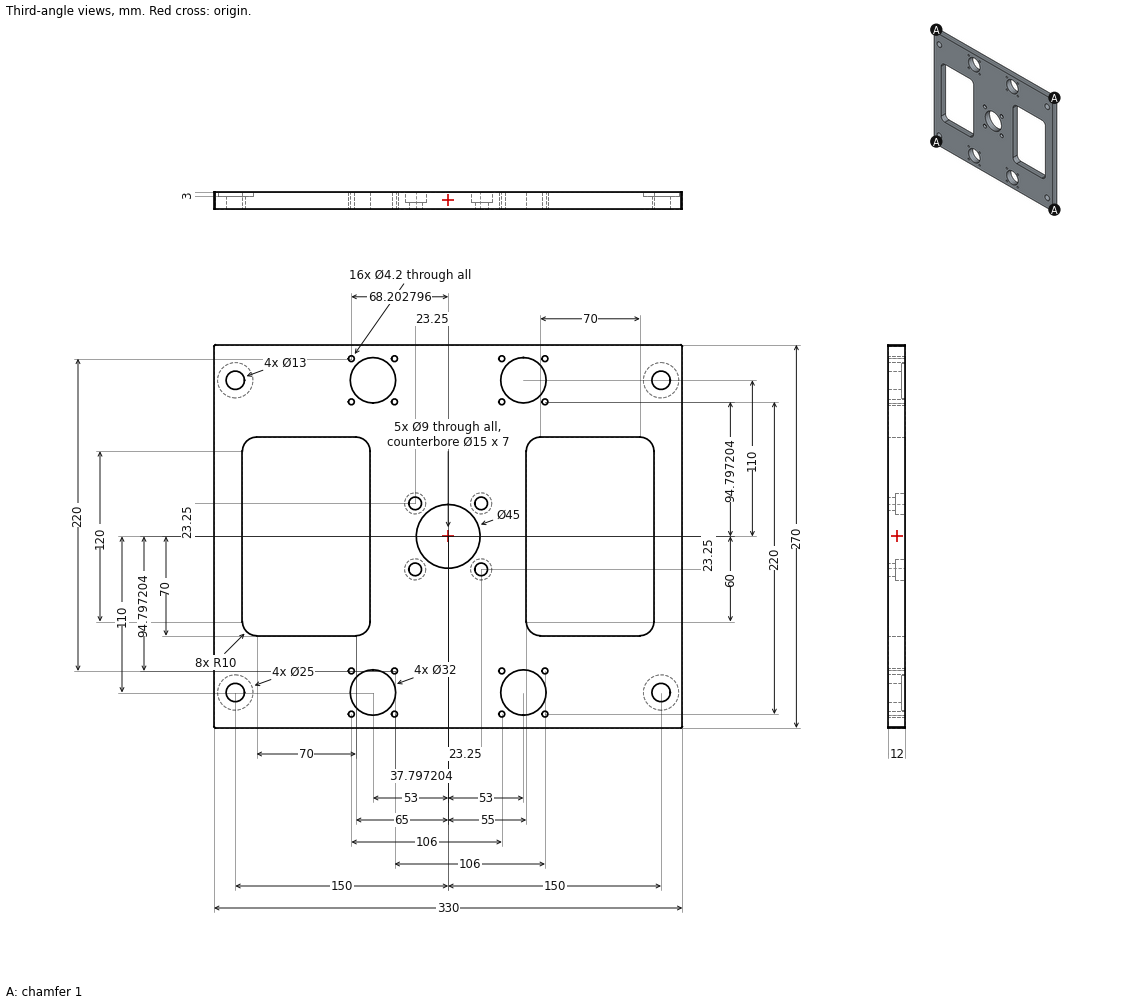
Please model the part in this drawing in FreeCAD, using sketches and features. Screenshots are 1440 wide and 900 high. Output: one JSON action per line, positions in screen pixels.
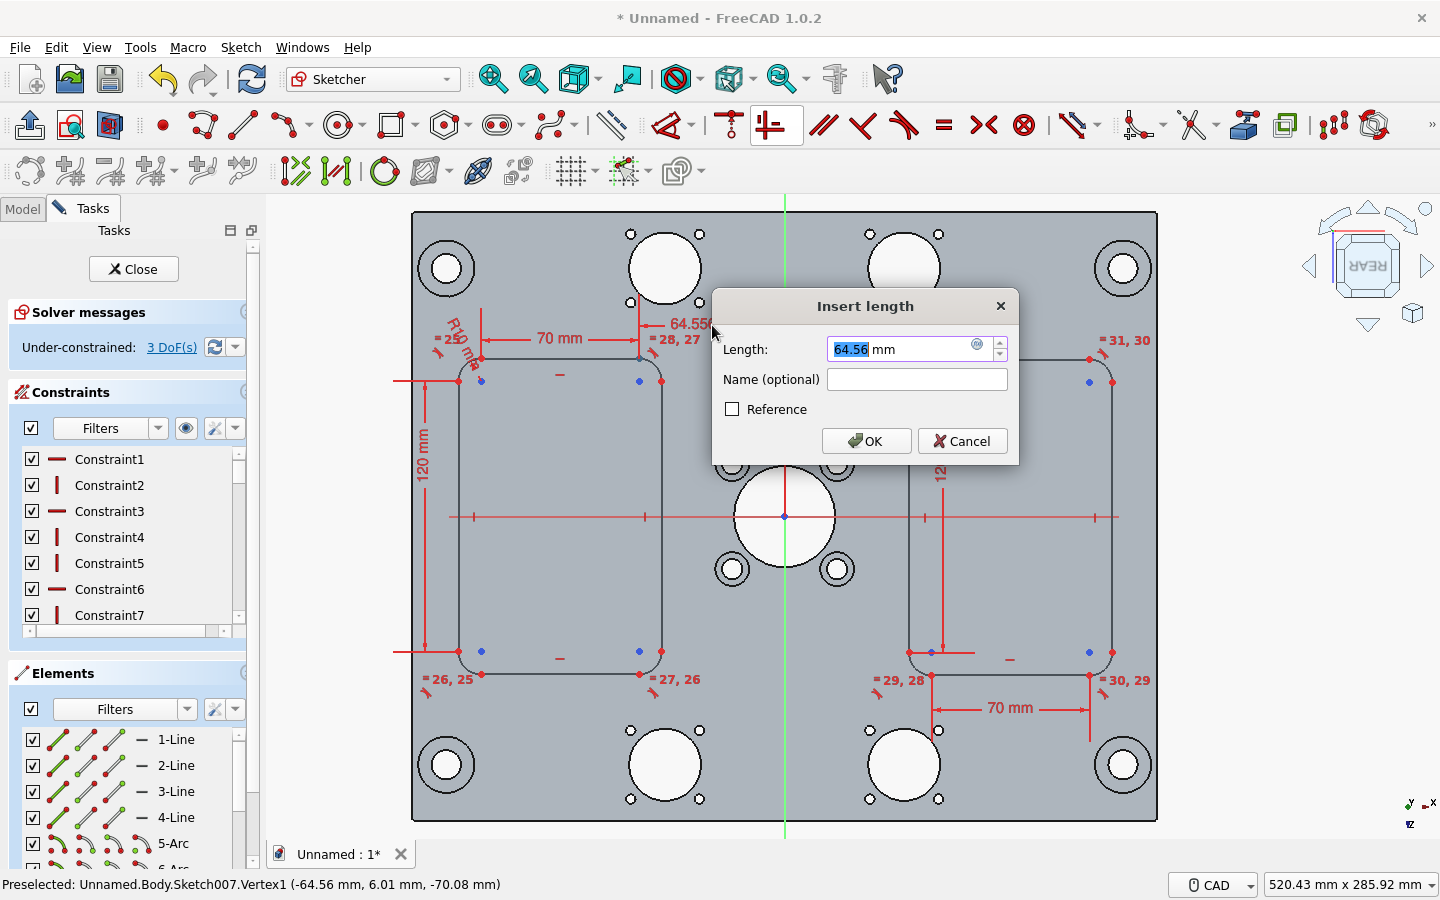
{"action": "type", "text": "65"}
{"action": "key", "text": "Return"}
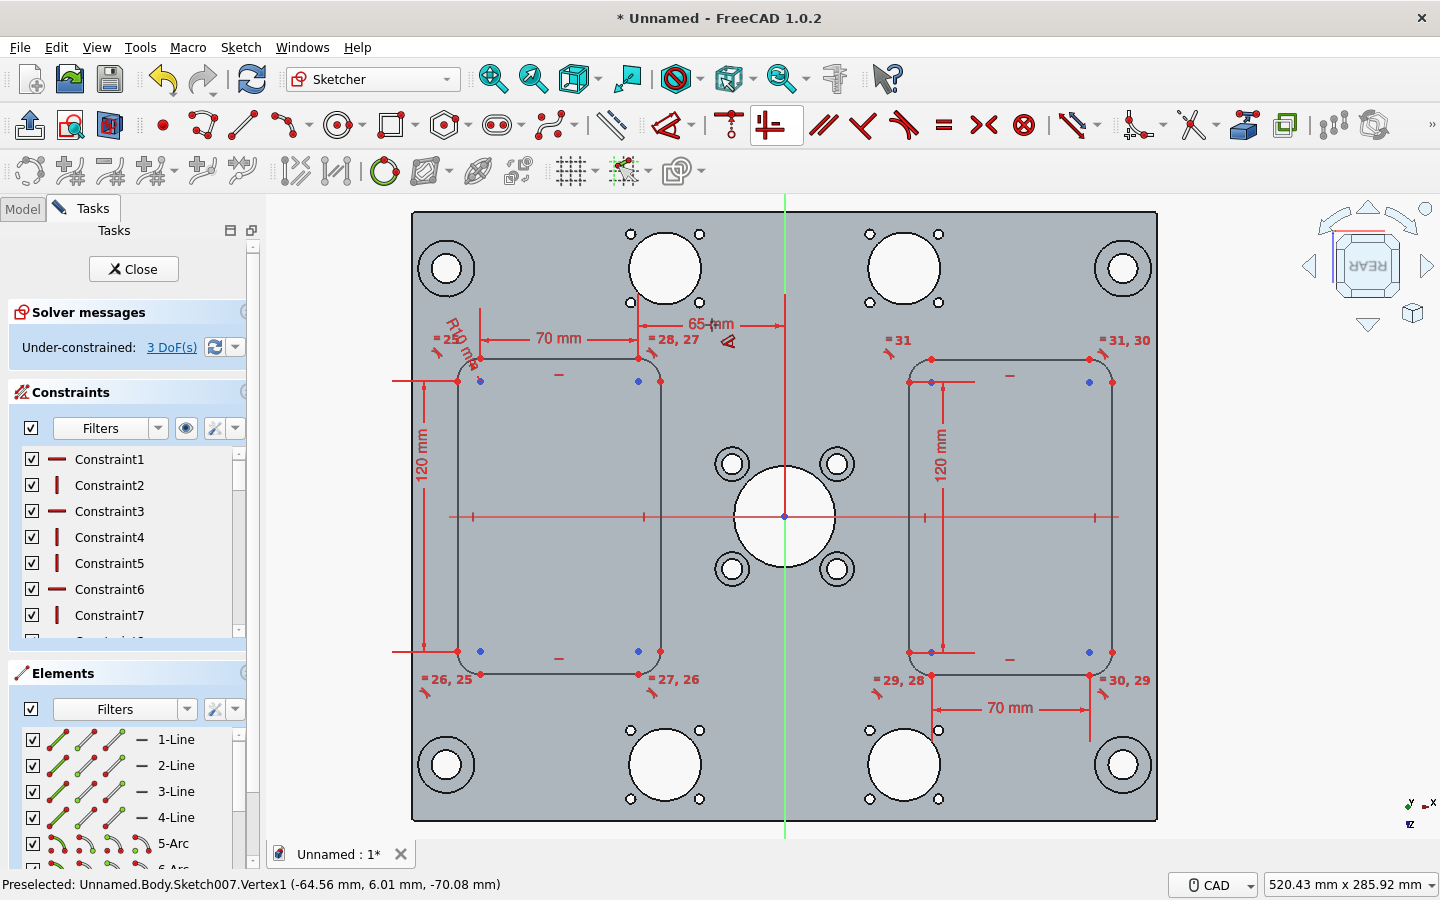
{"action": "left_click", "coordinate": [638, 359]}
{"action": "left_click", "coordinate": [604, 438]}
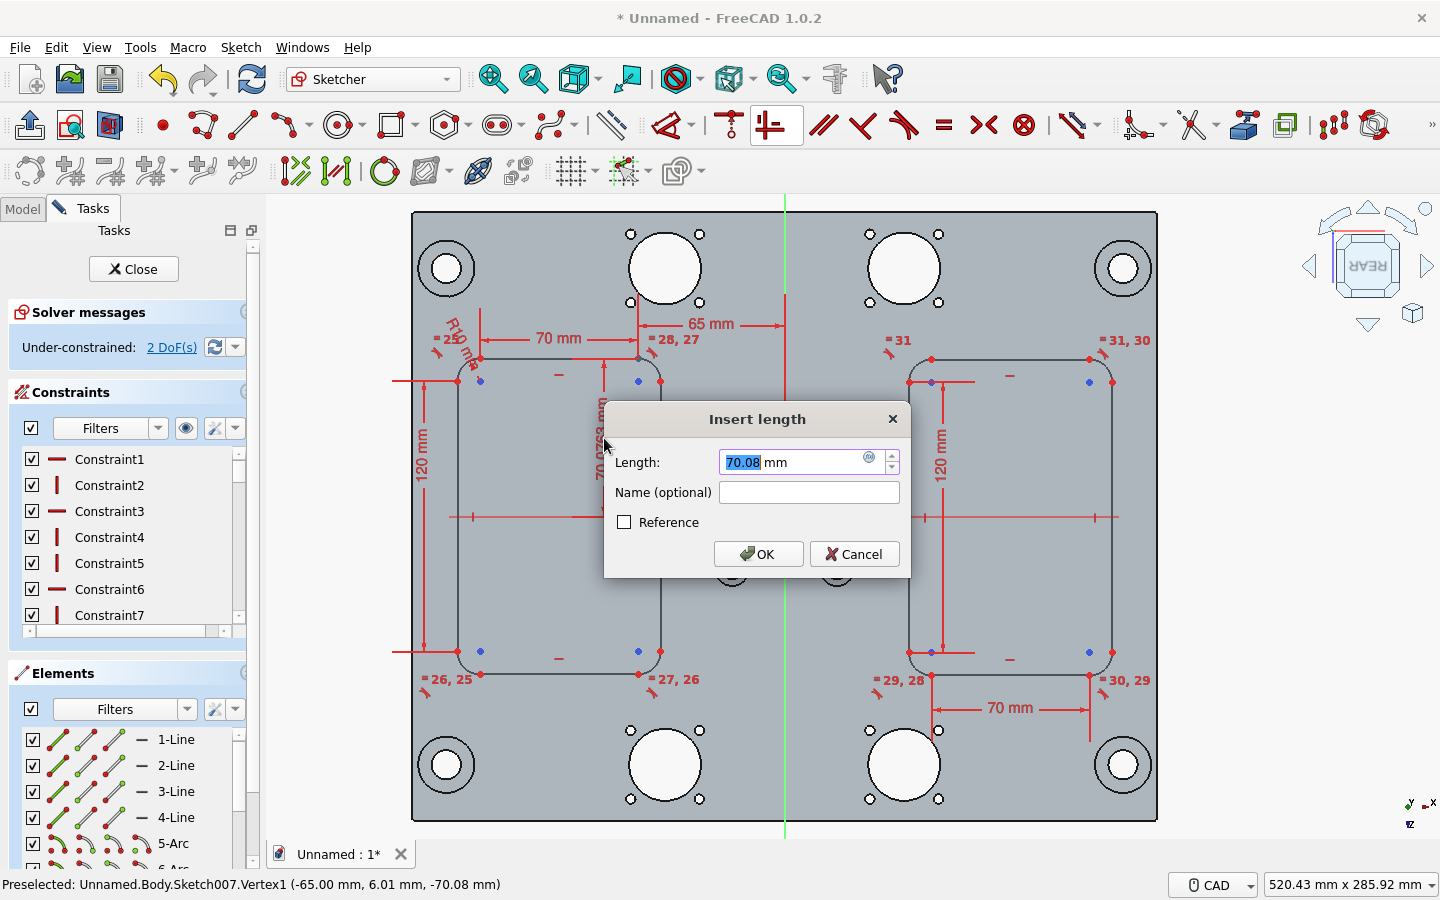
{"action": "type", "text": "70"}
{"action": "key", "text": "Return"}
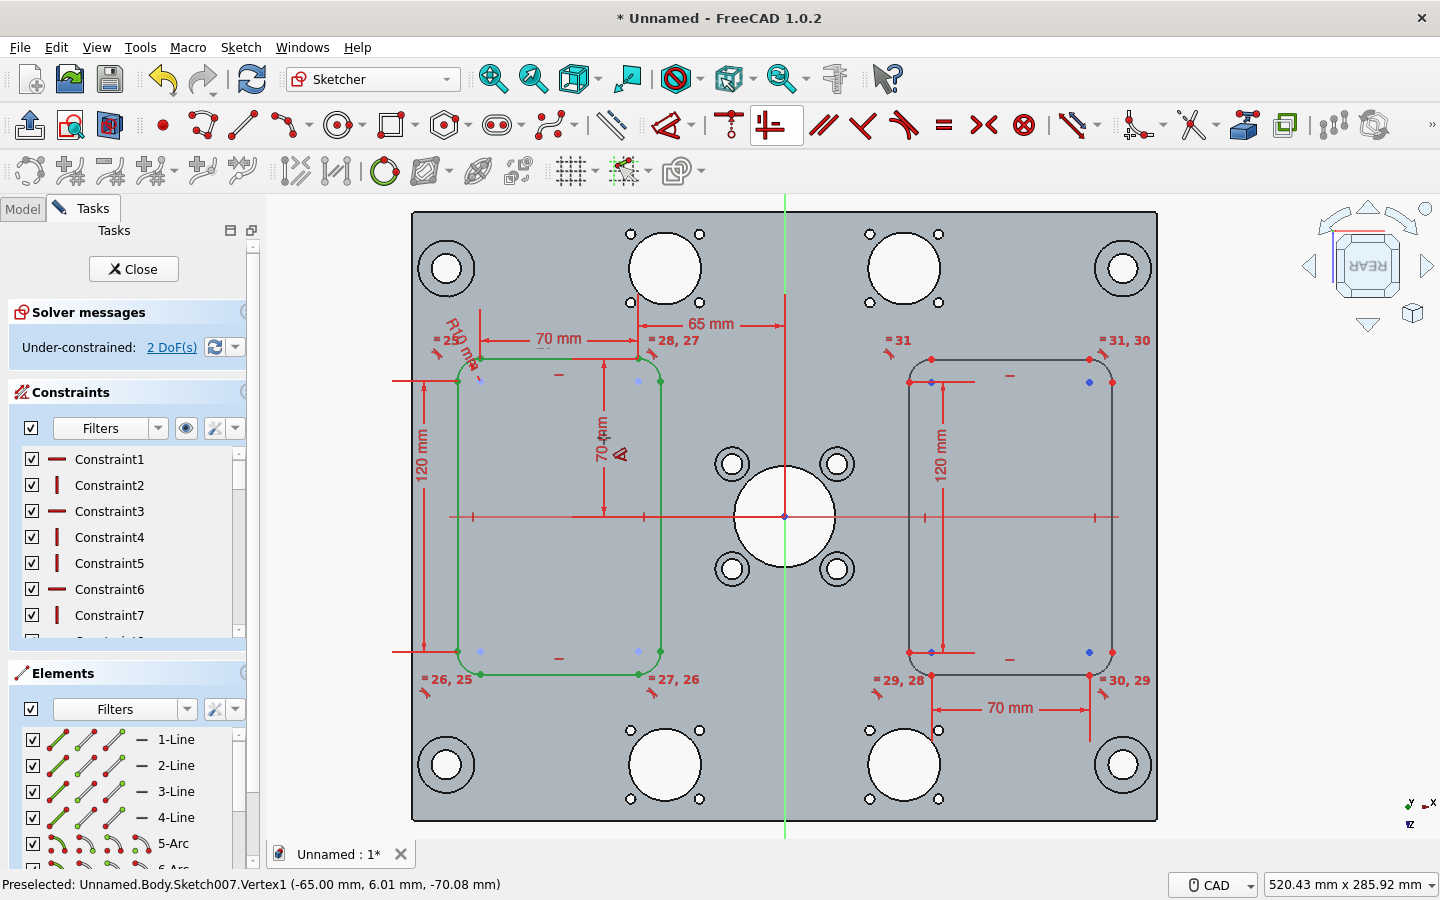
{"action": "left_click", "coordinate": [909, 382]}
{"action": "left_click", "coordinate": [847, 348]}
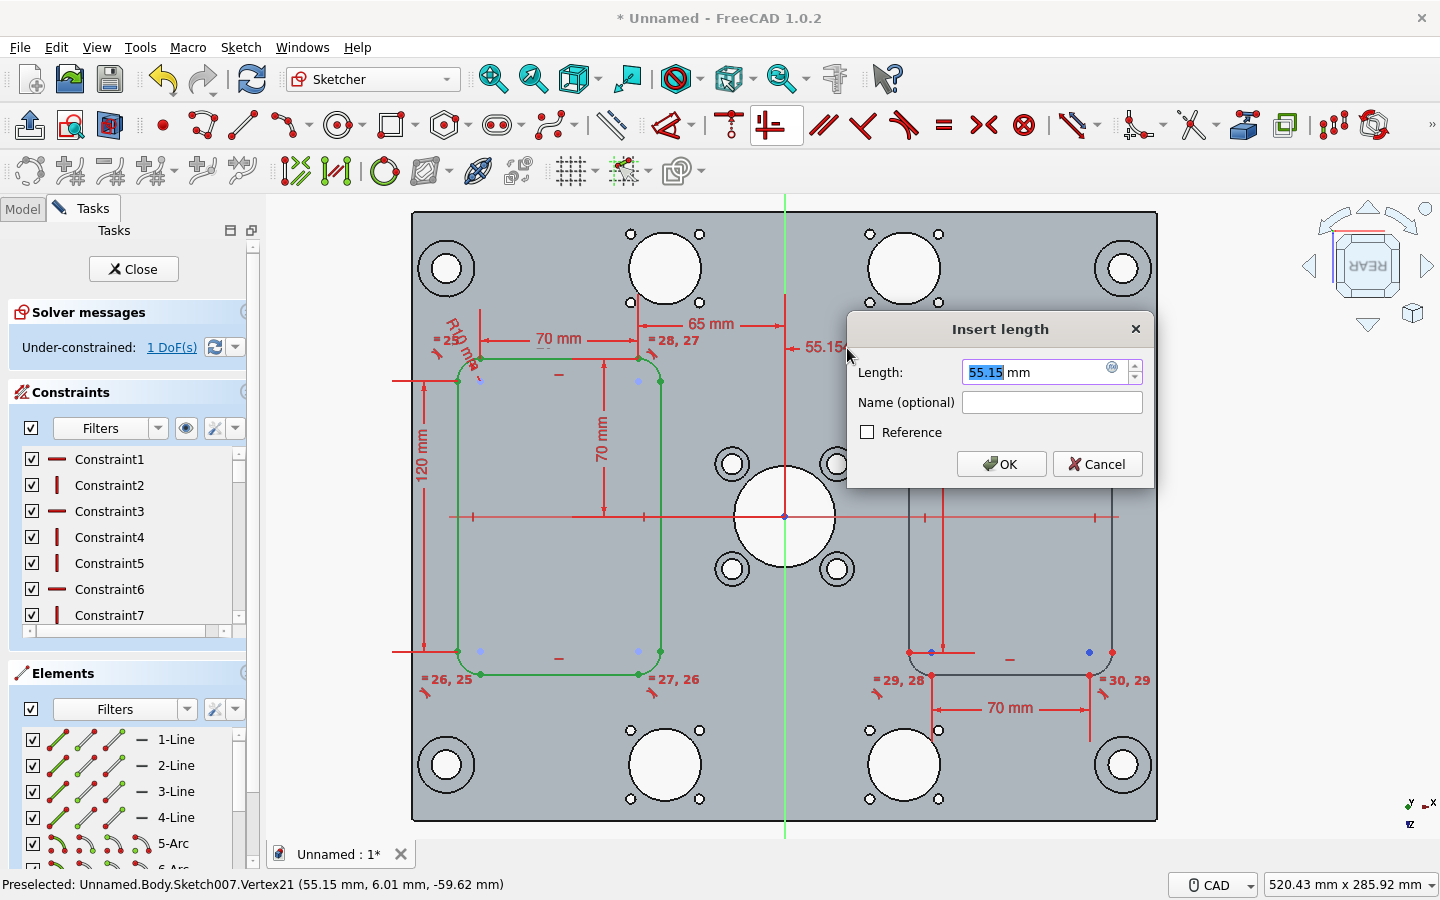
{"action": "type", "text": "55"}
{"action": "key", "text": "Return"}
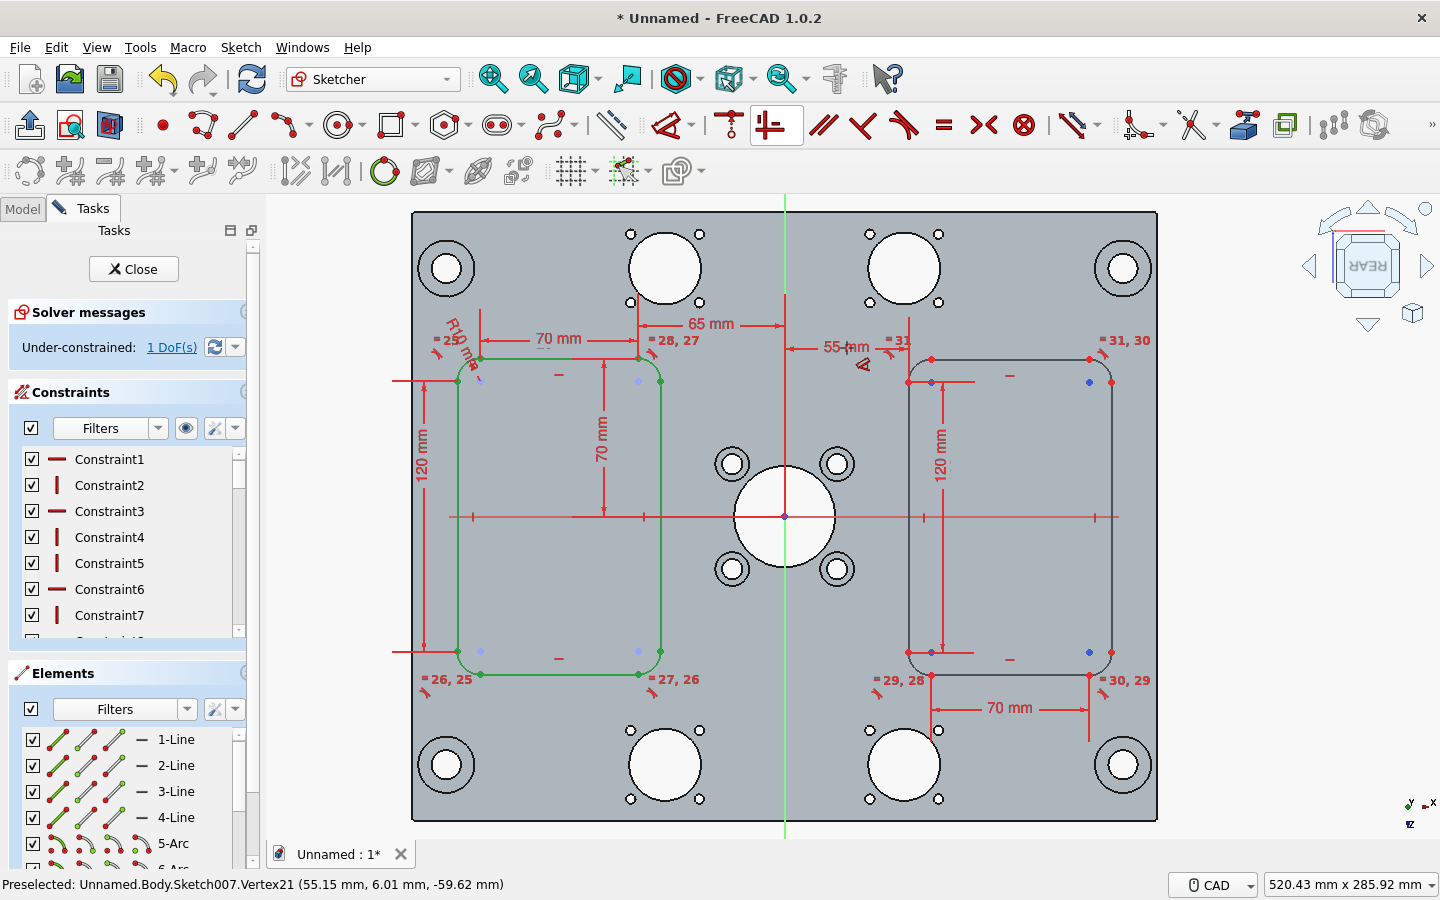
{"action": "left_click", "coordinate": [909, 382]}
{"action": "left_click", "coordinate": [943, 418]}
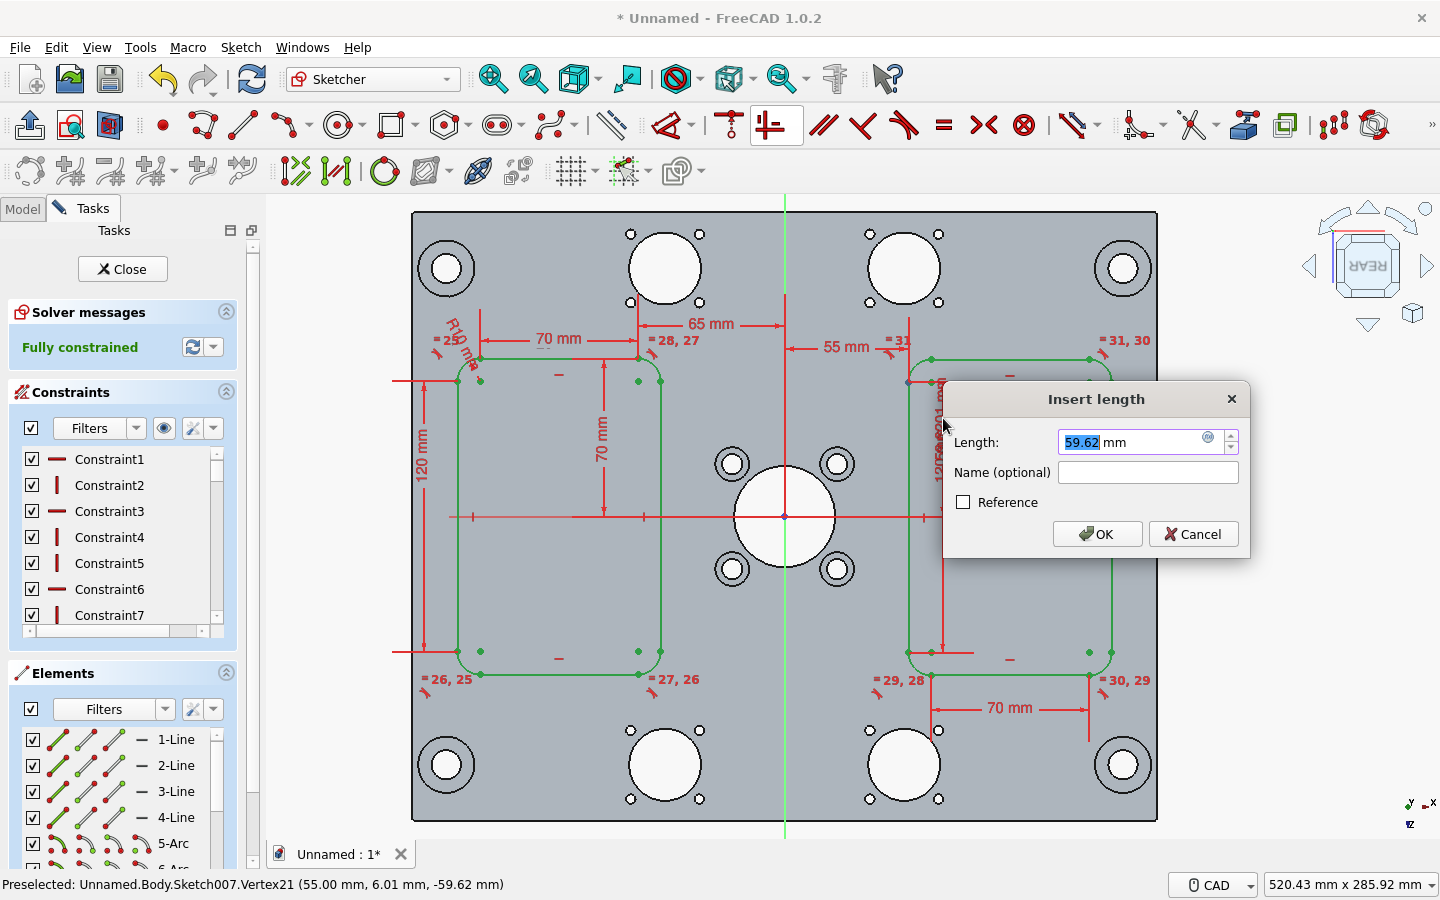
{"action": "type", "text": "60"}
{"action": "key", "text": "Return"}
{"action": "key", "text": "Escape"}